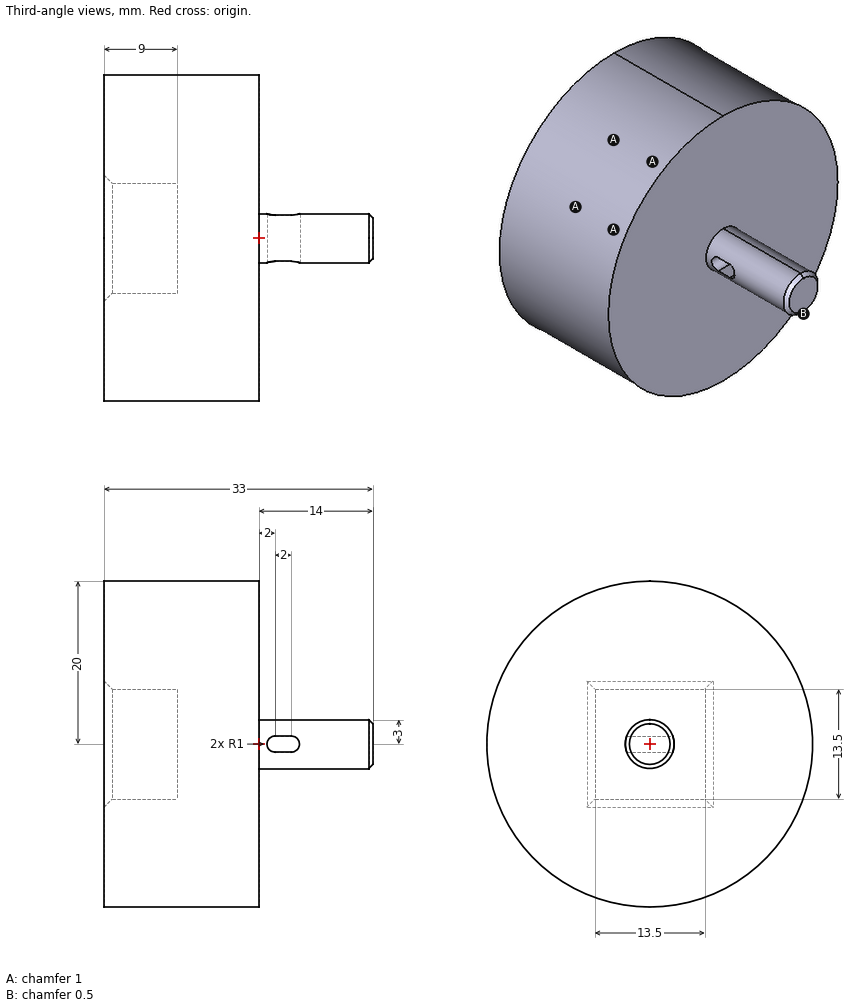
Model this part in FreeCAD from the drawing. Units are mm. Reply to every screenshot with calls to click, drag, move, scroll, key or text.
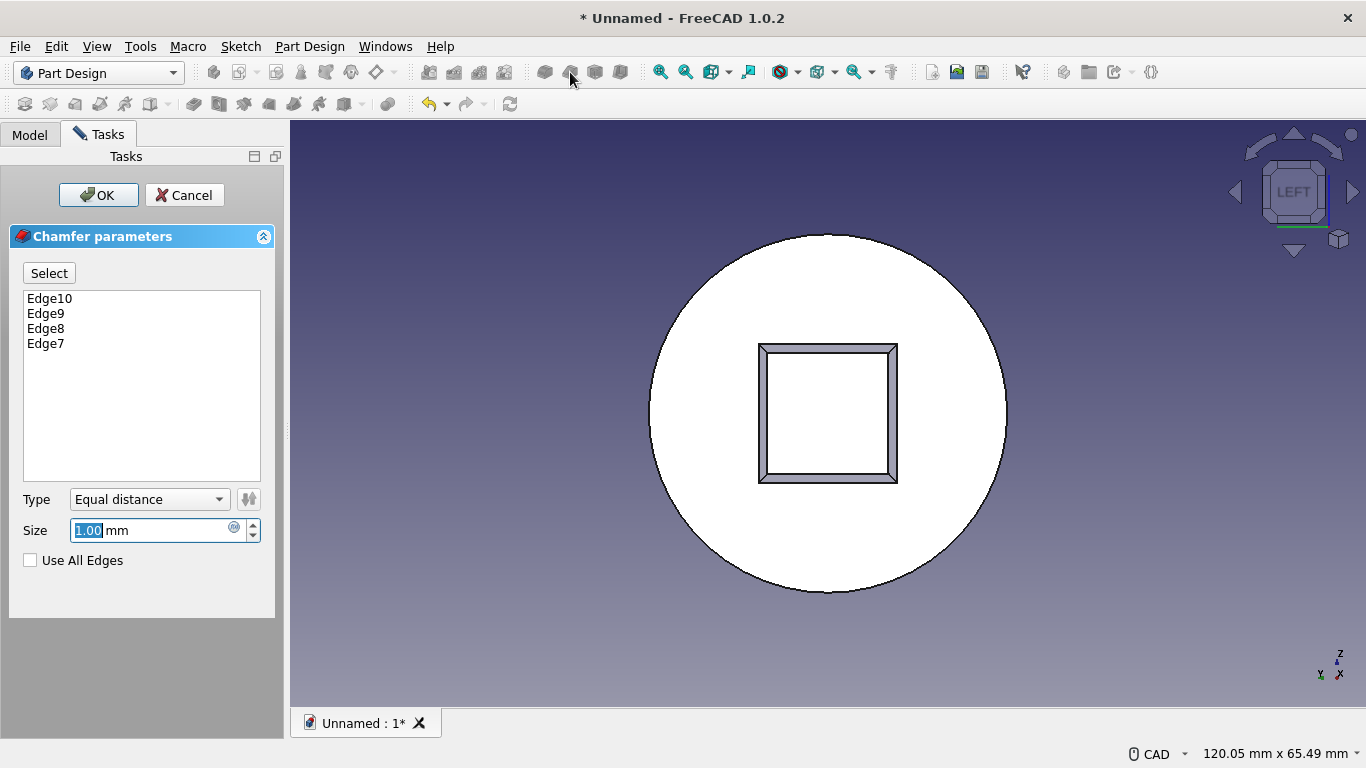
text(1)
key(Tab)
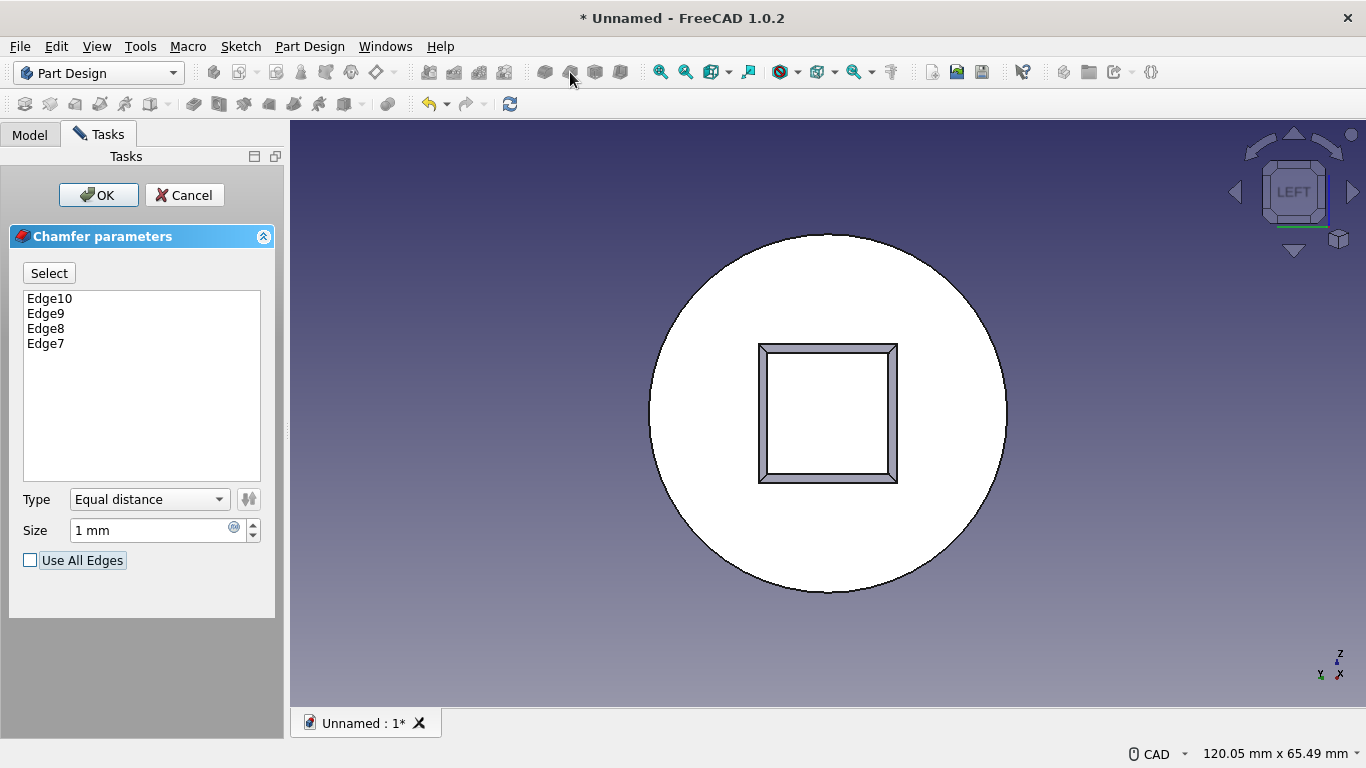
click(99, 195)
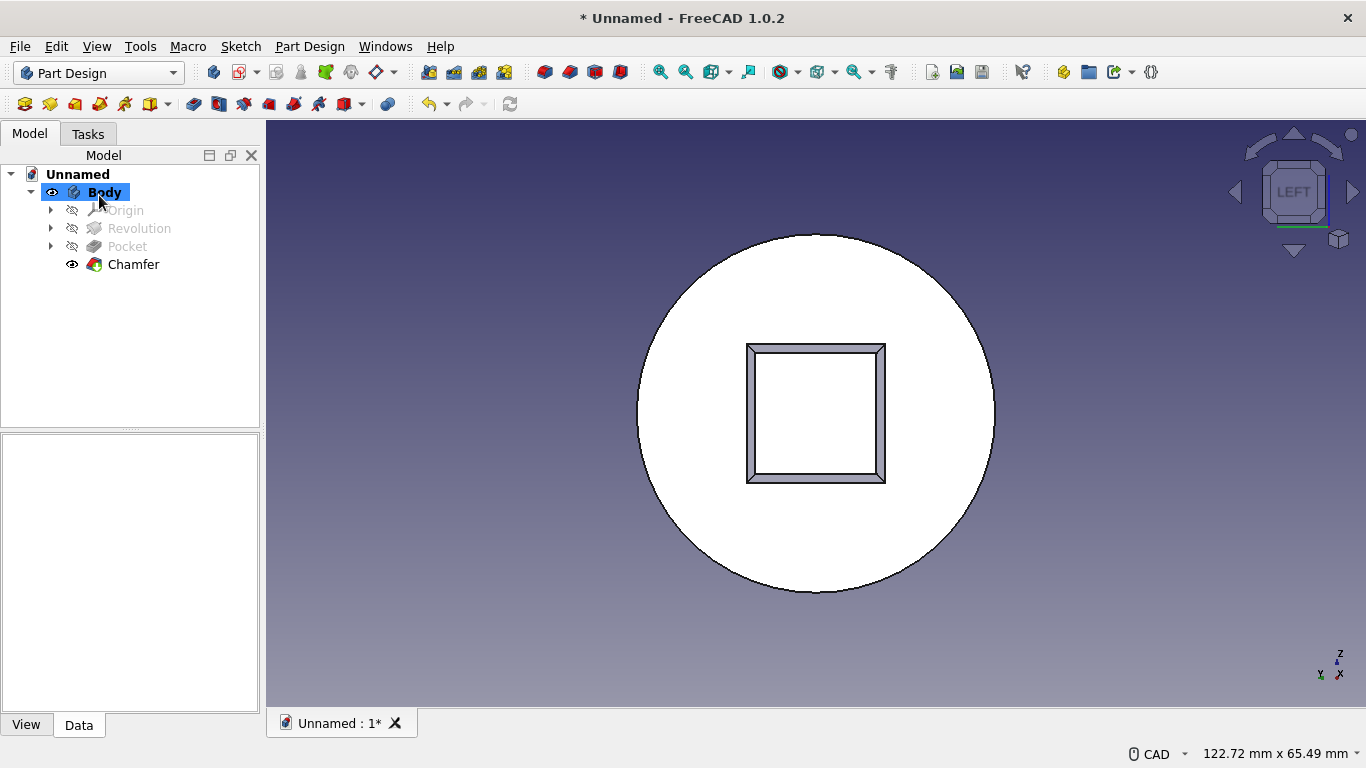
click(238, 72)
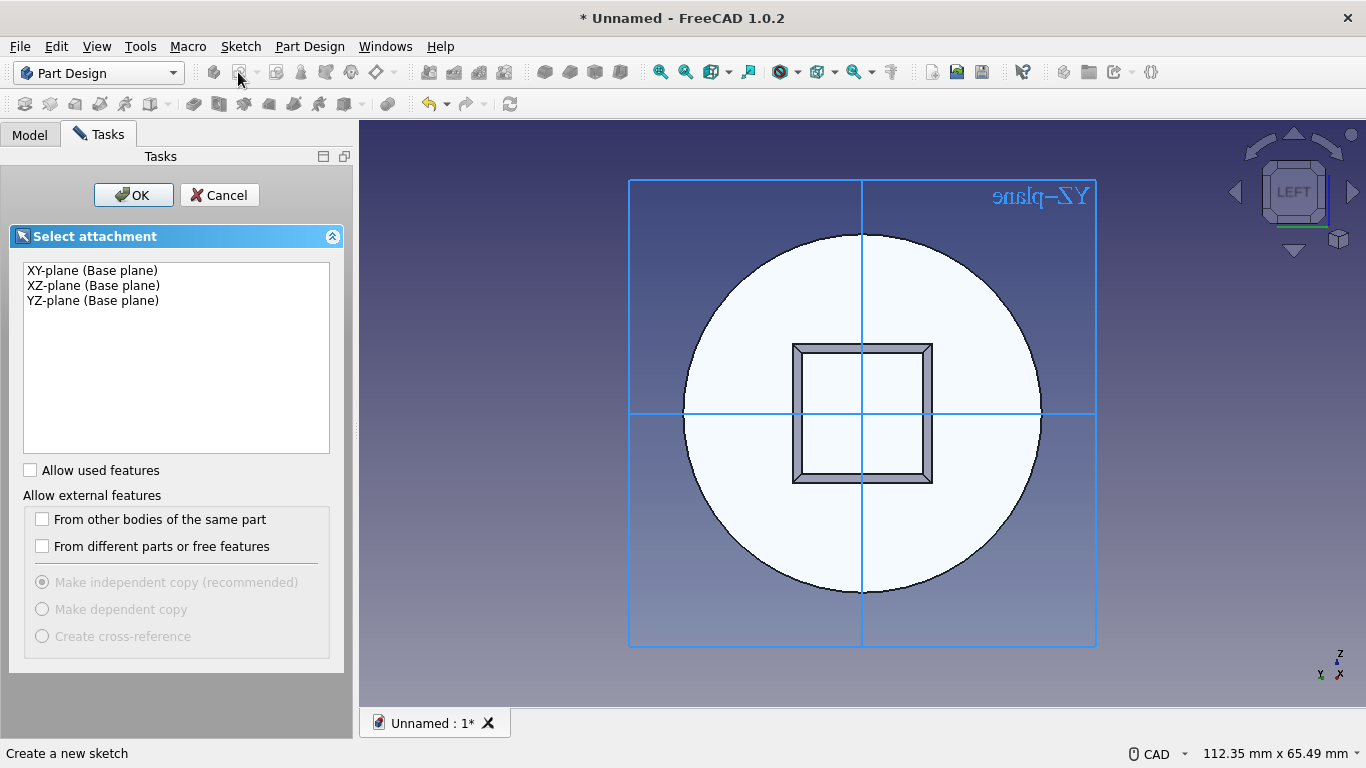
click(84, 286)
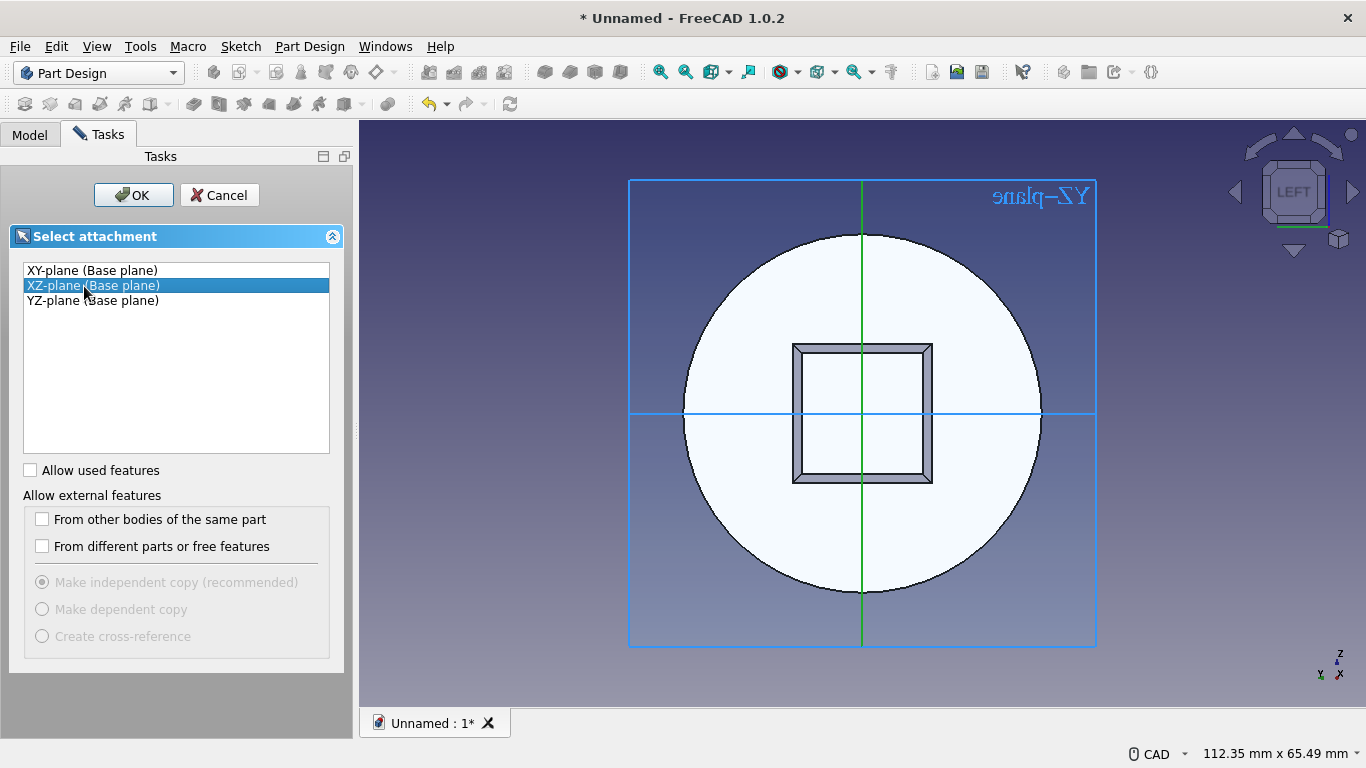
click(134, 195)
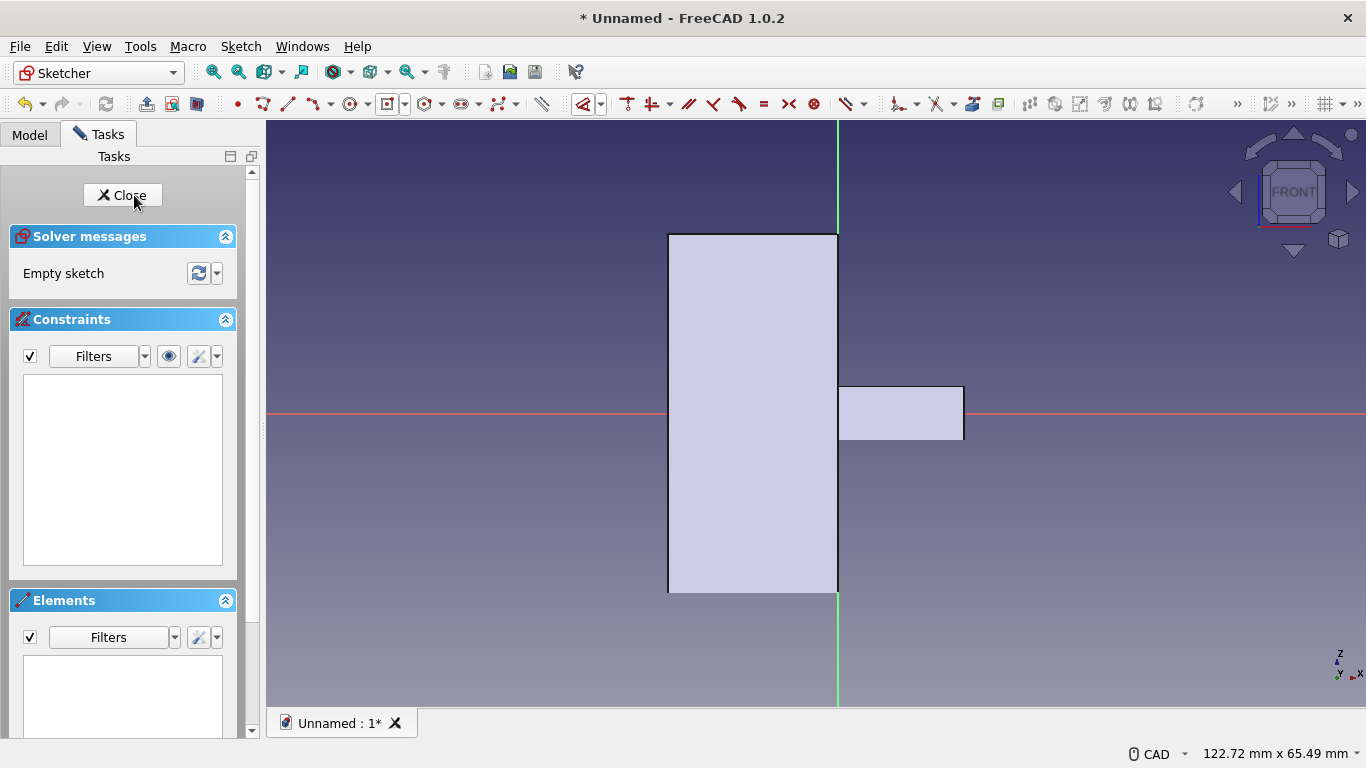
click(197, 104)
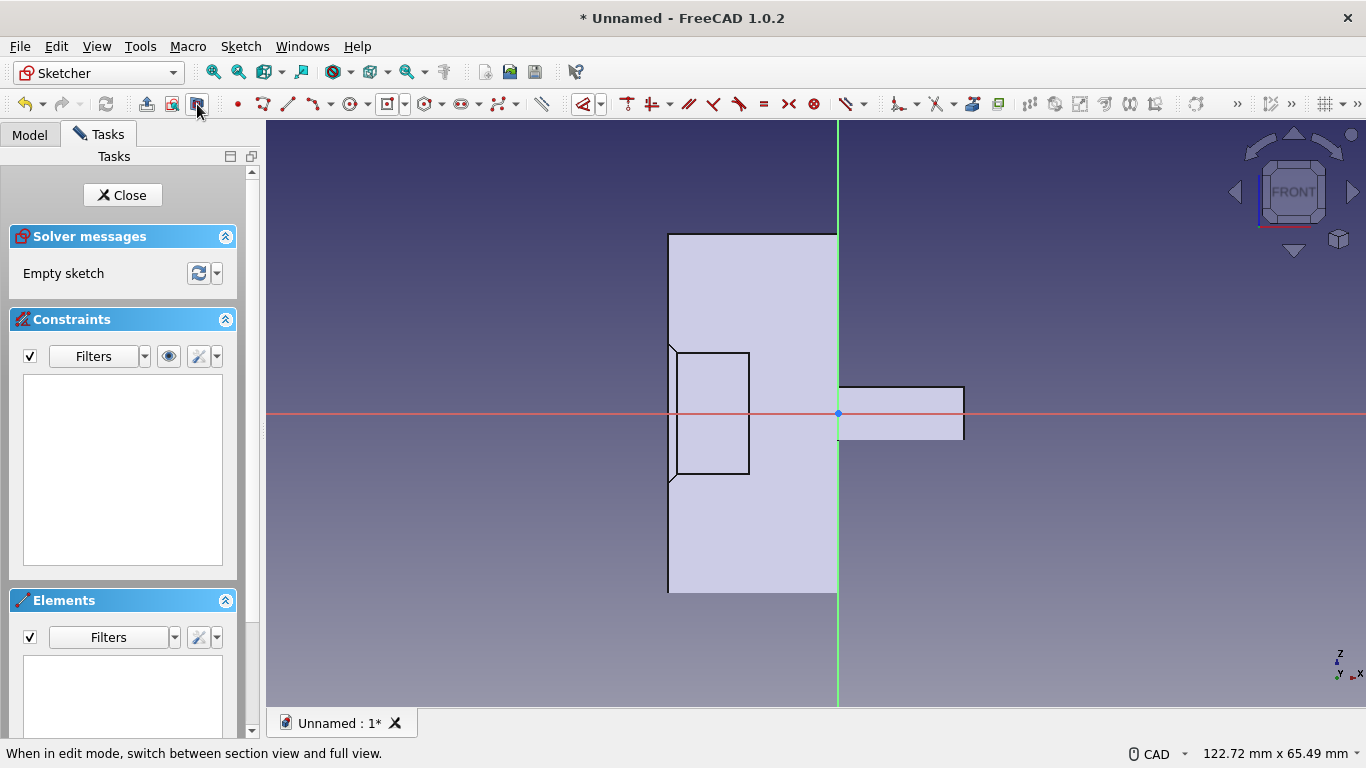
scroll(870, 414, up, 13)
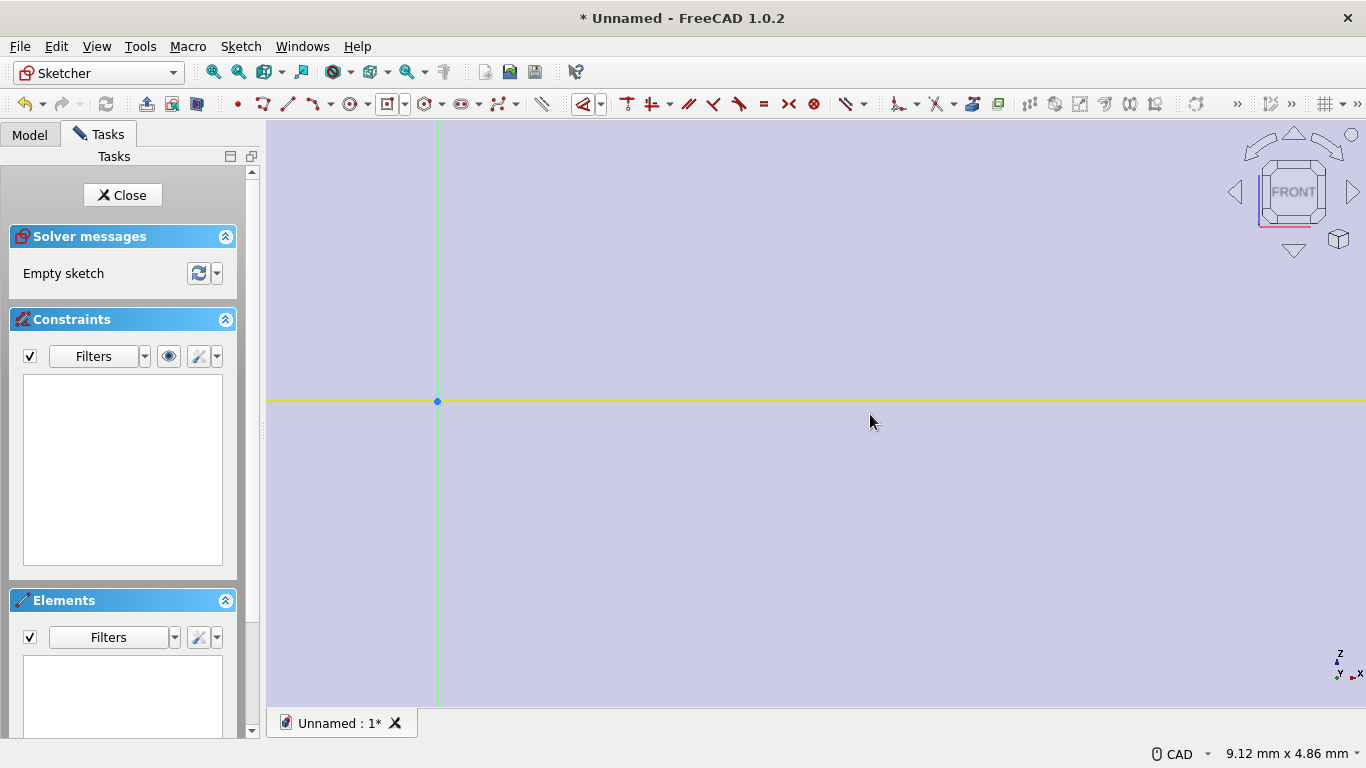
click(460, 104)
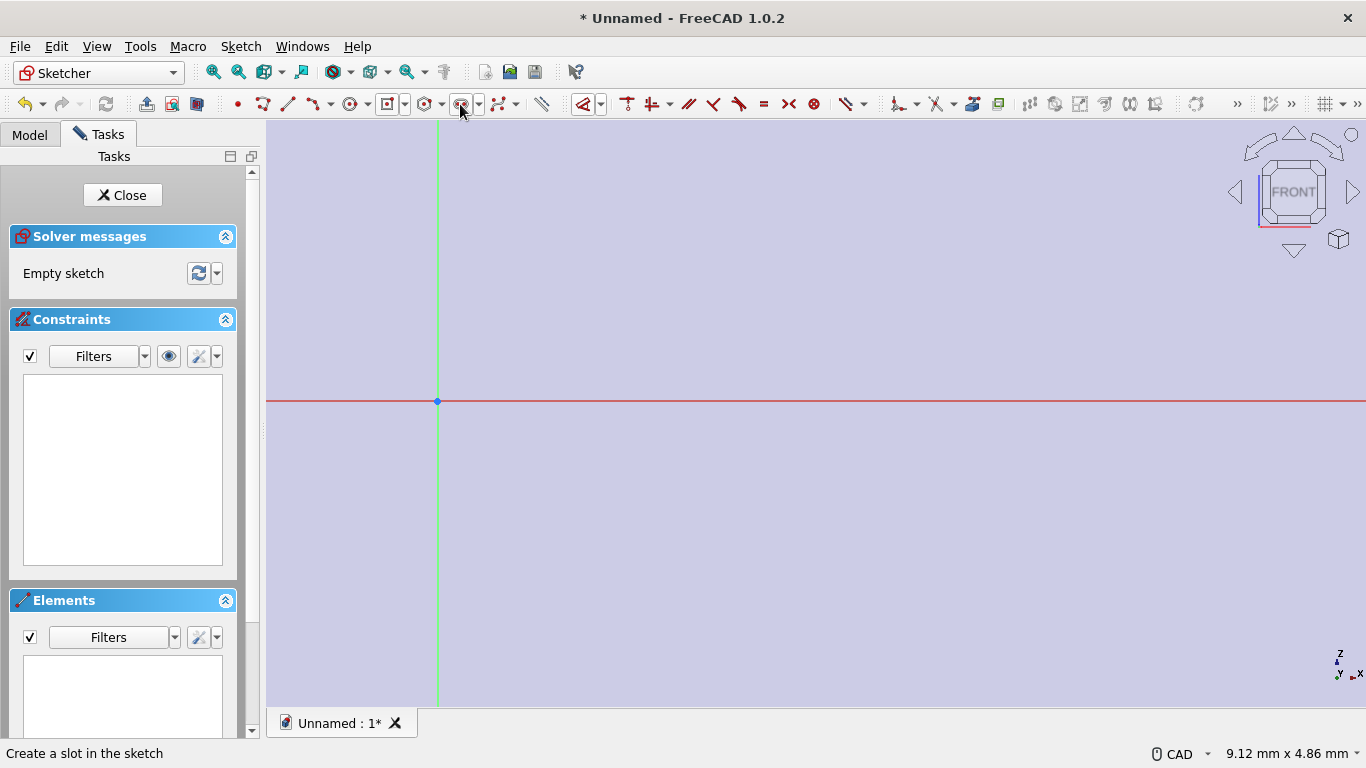
click(679, 401)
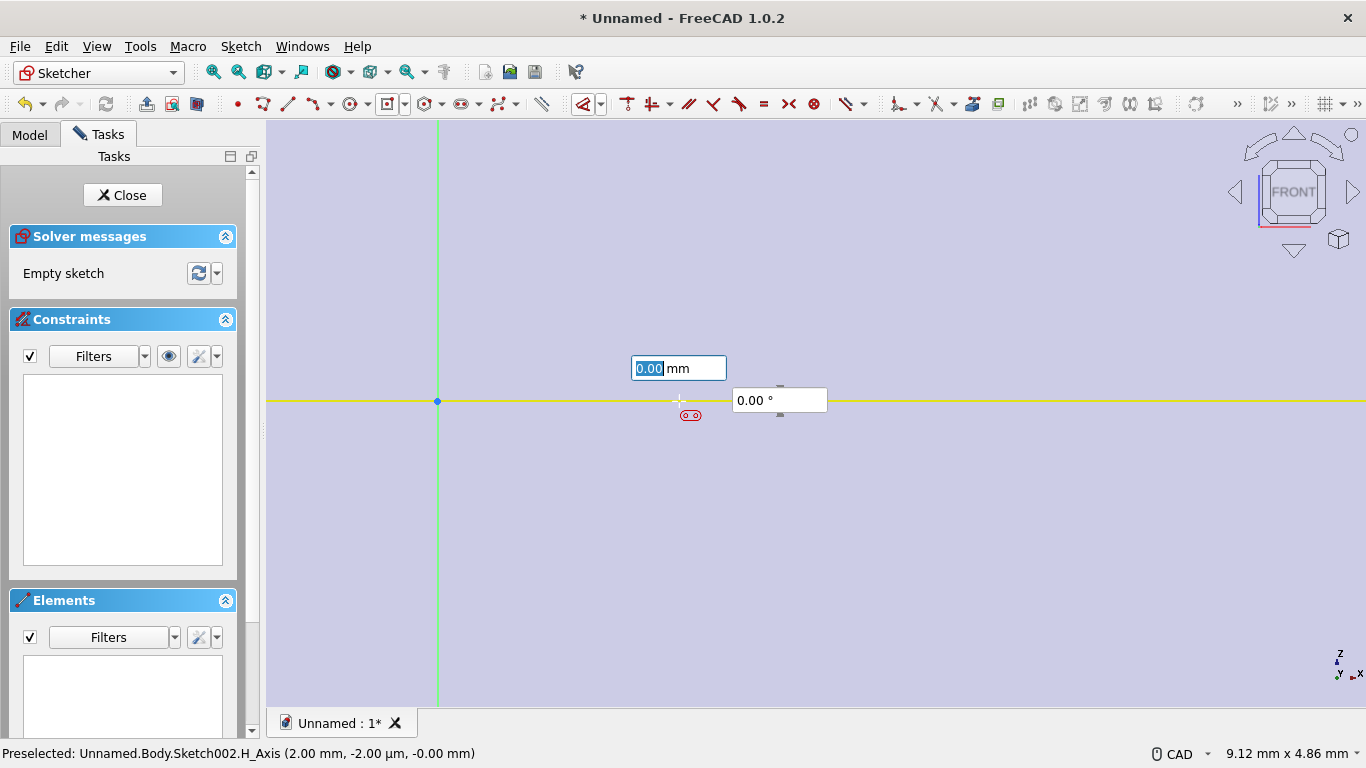
click(921, 392)